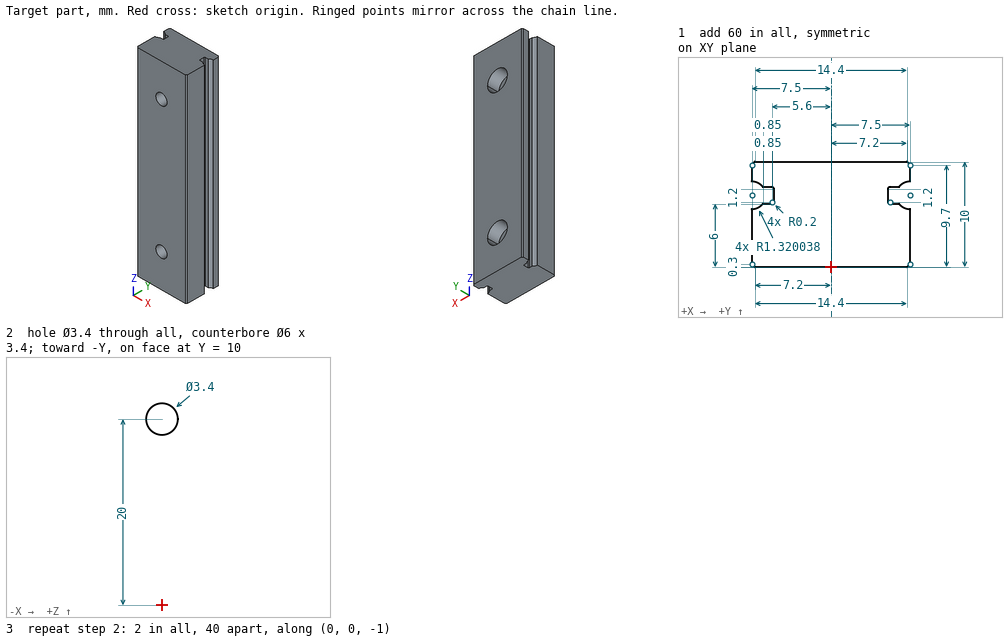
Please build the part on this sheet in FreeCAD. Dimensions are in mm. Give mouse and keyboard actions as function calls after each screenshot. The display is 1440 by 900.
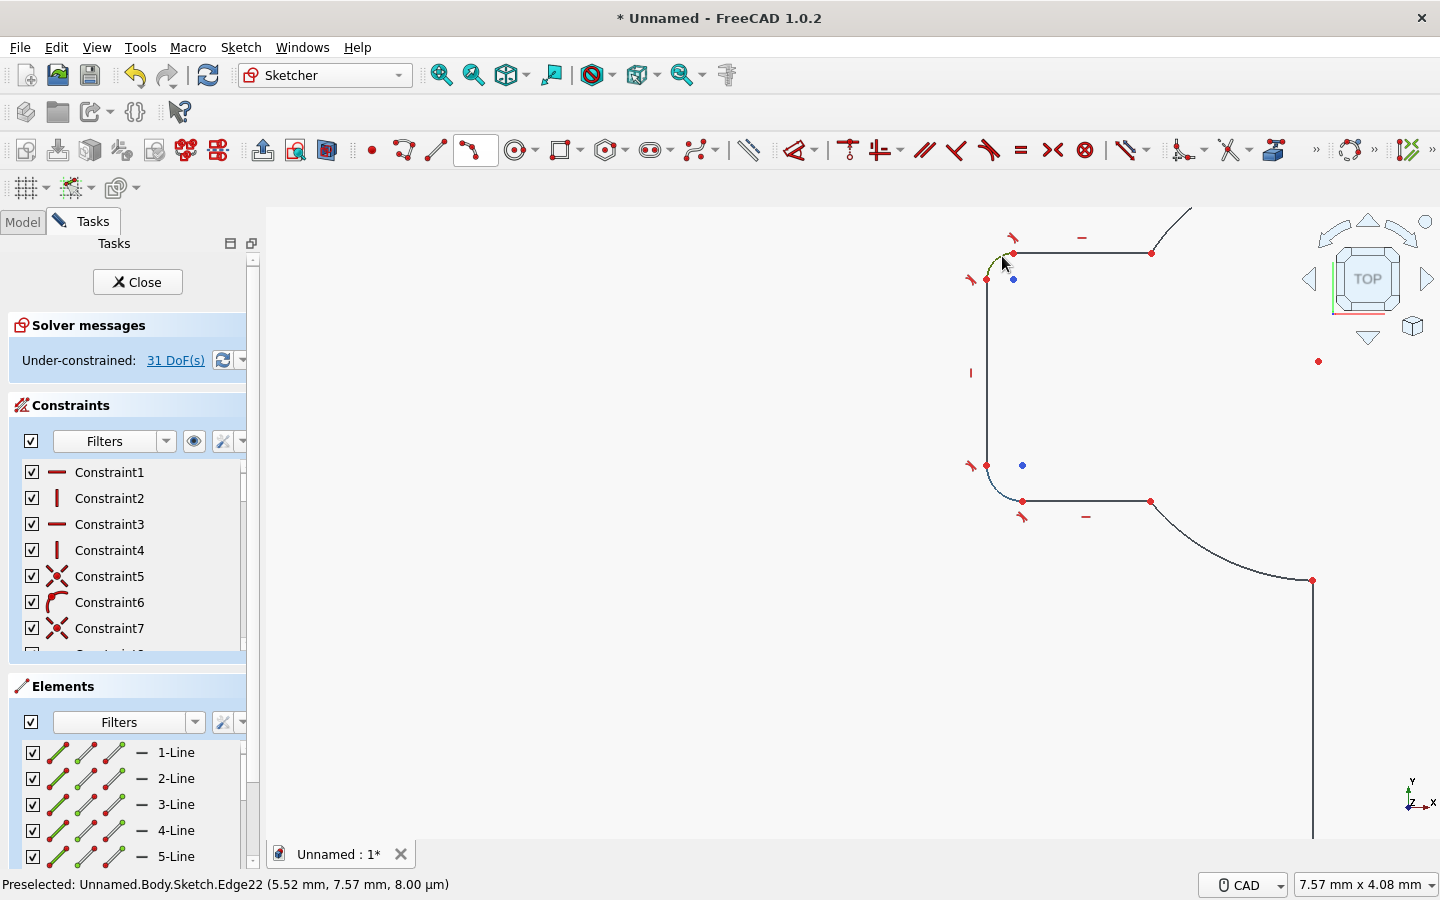
key(e)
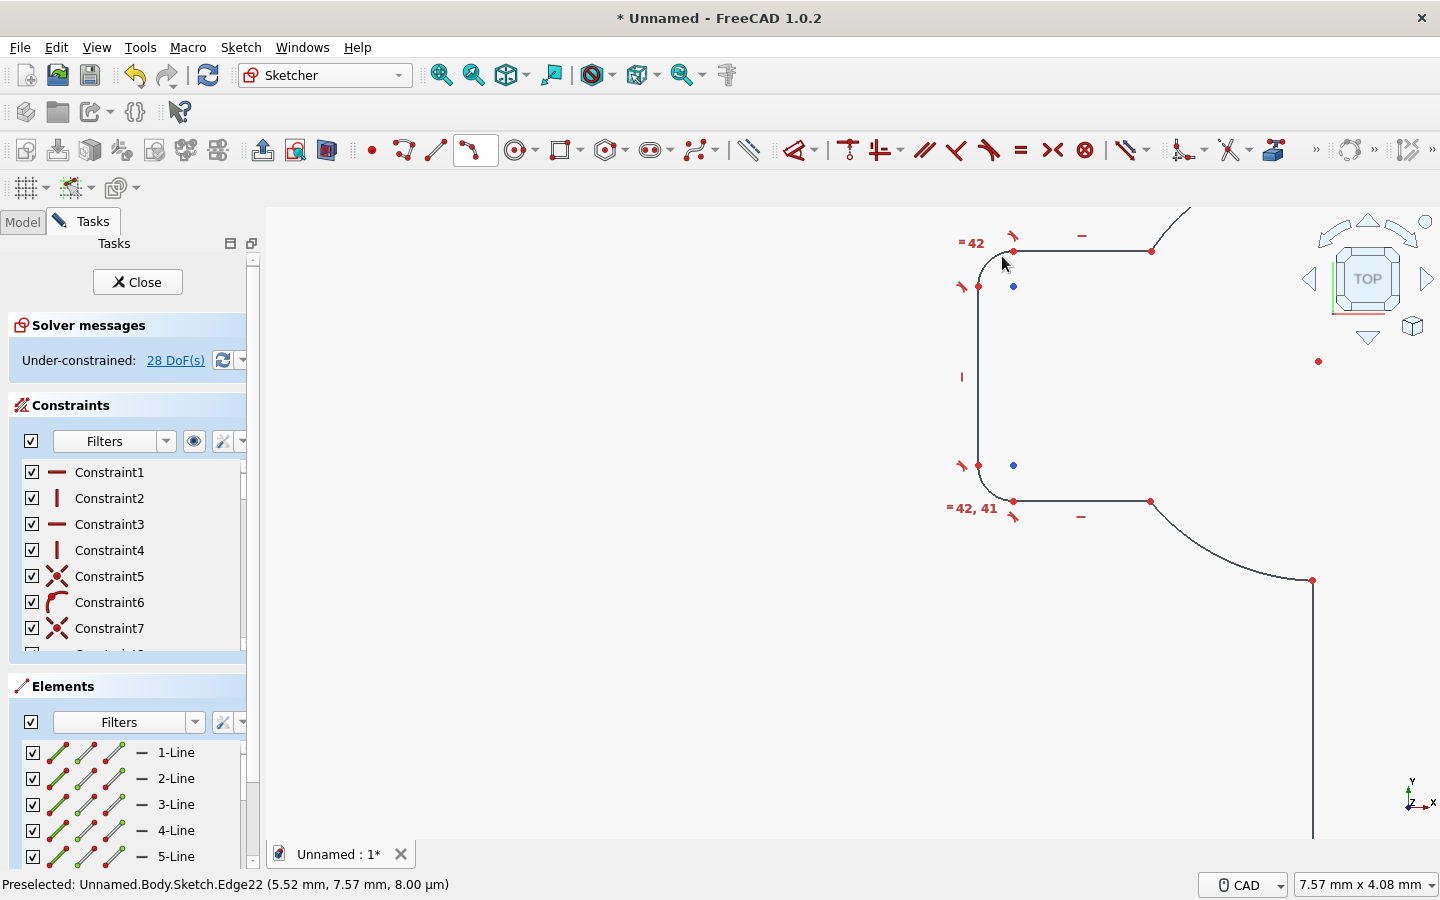
scroll(992, 481, down, 7)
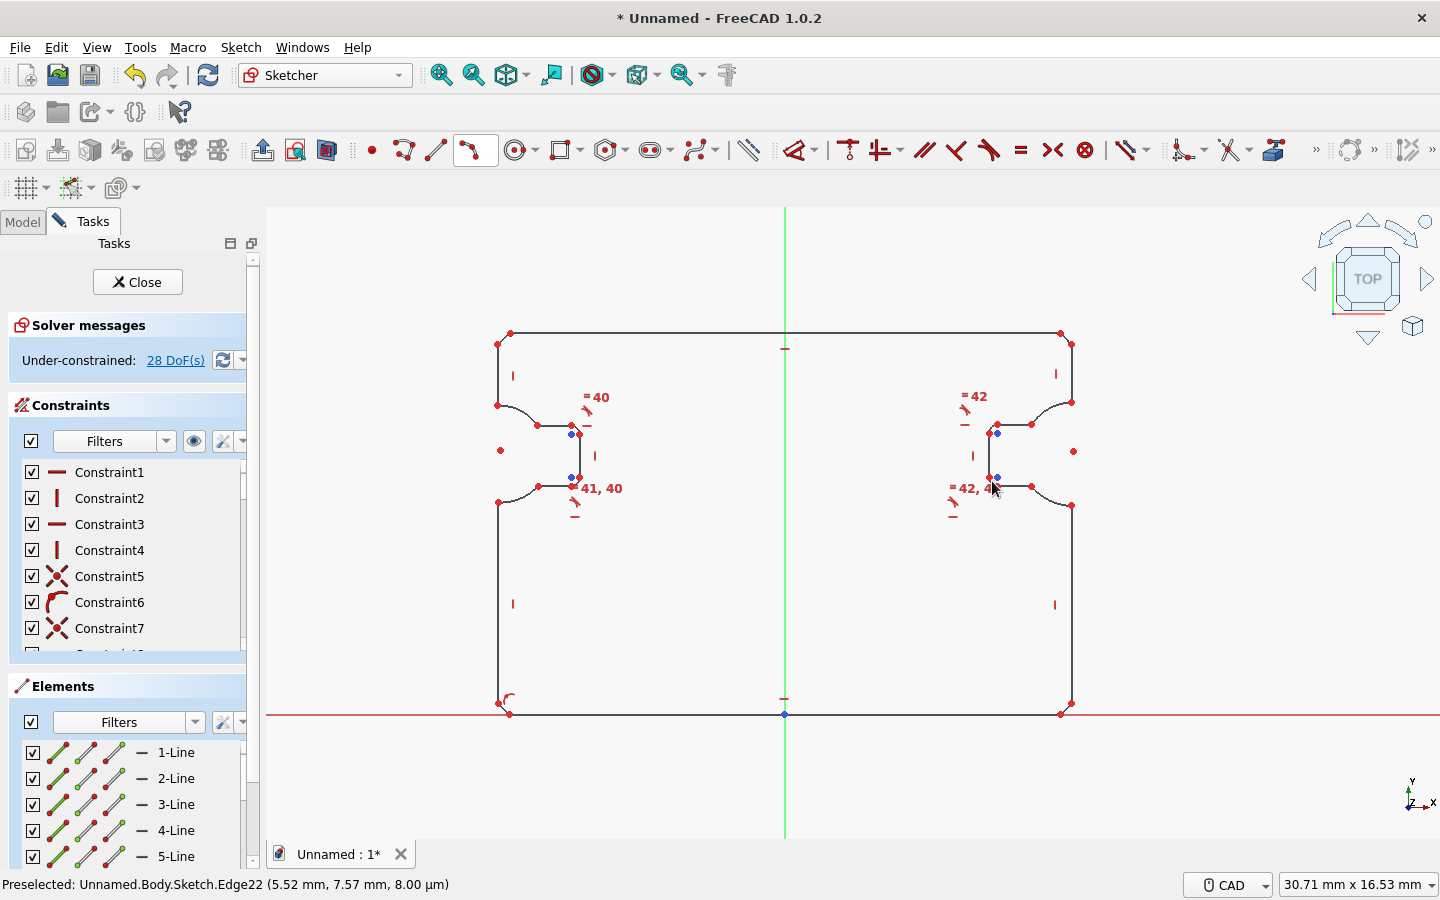
click(511, 501)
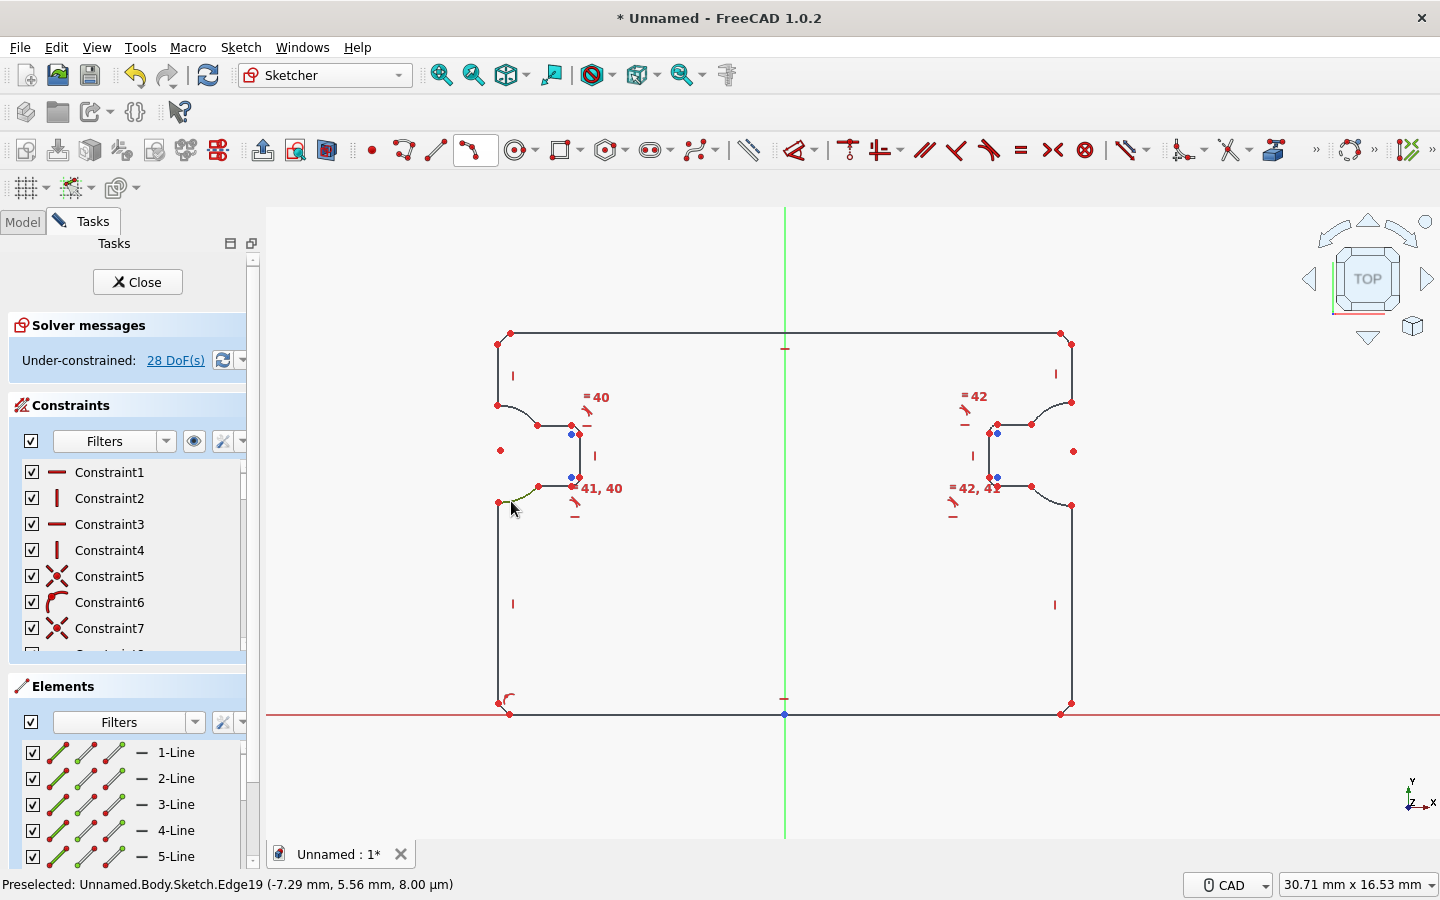
click(1041, 496)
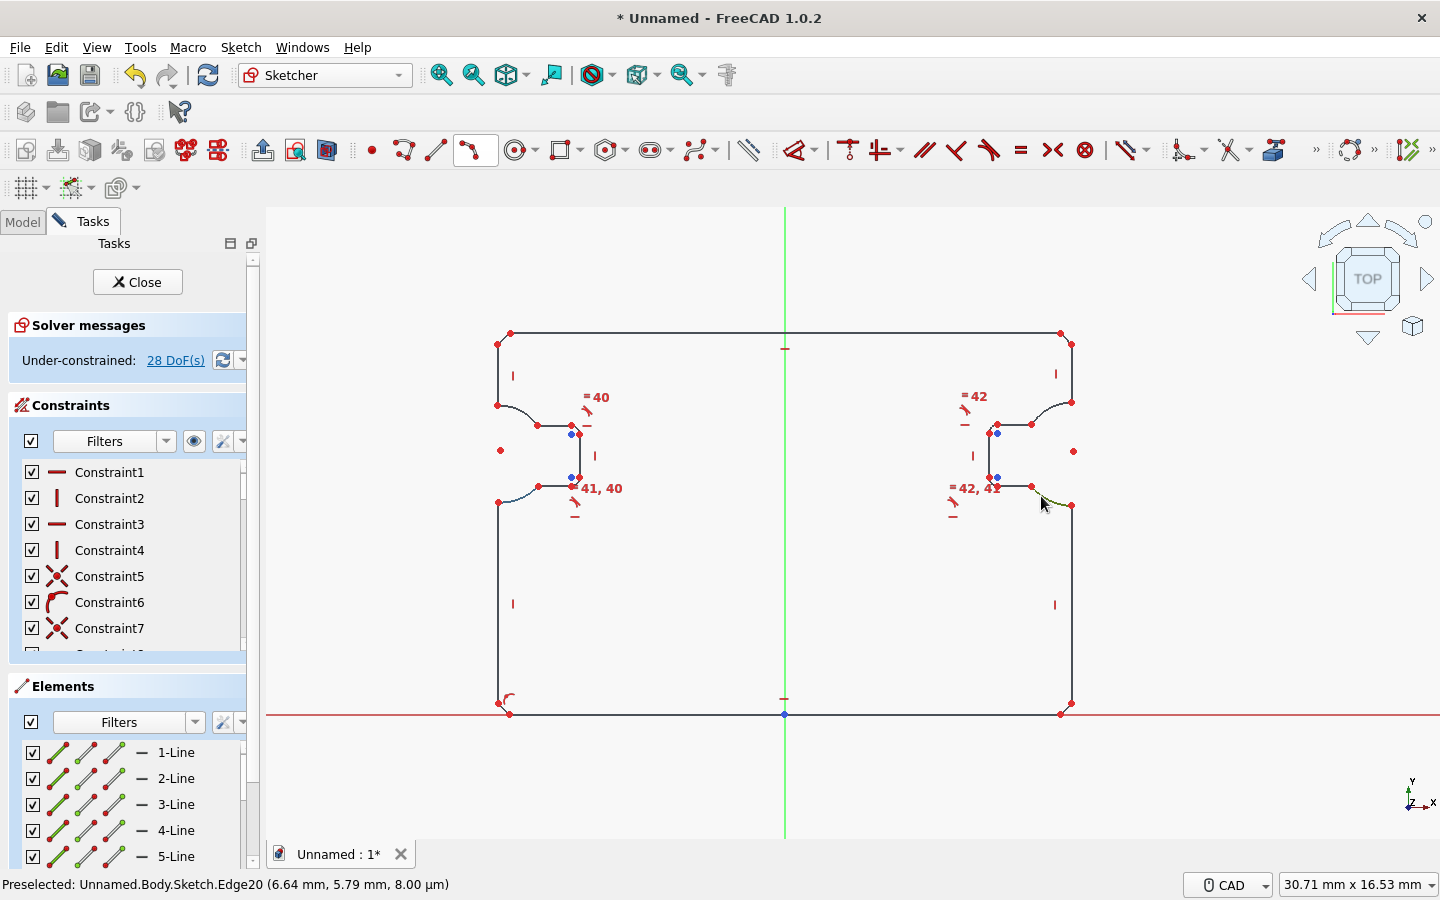
click(1058, 405)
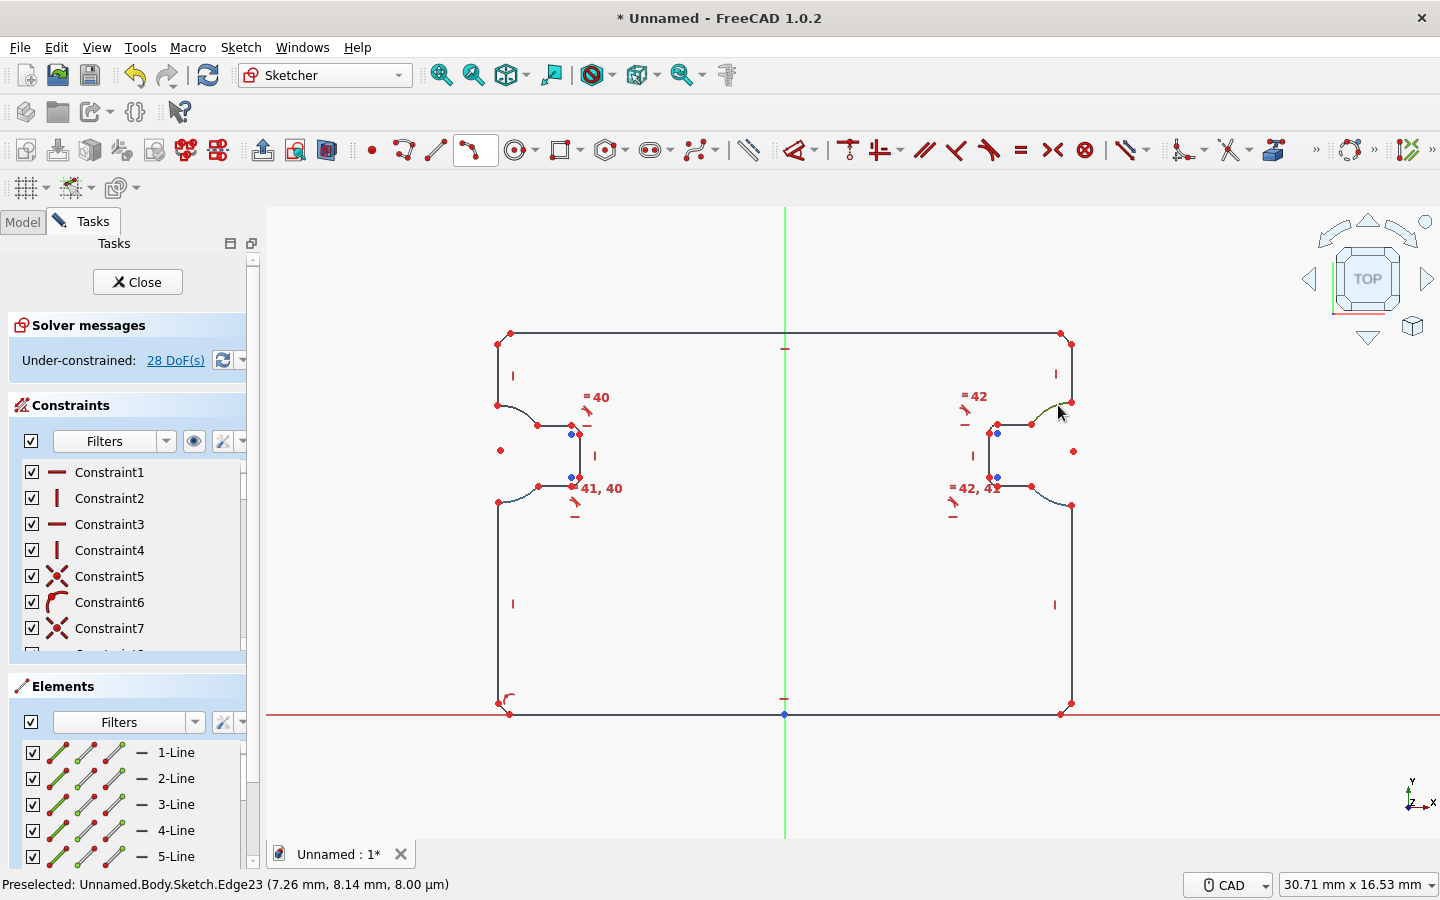
click(528, 415)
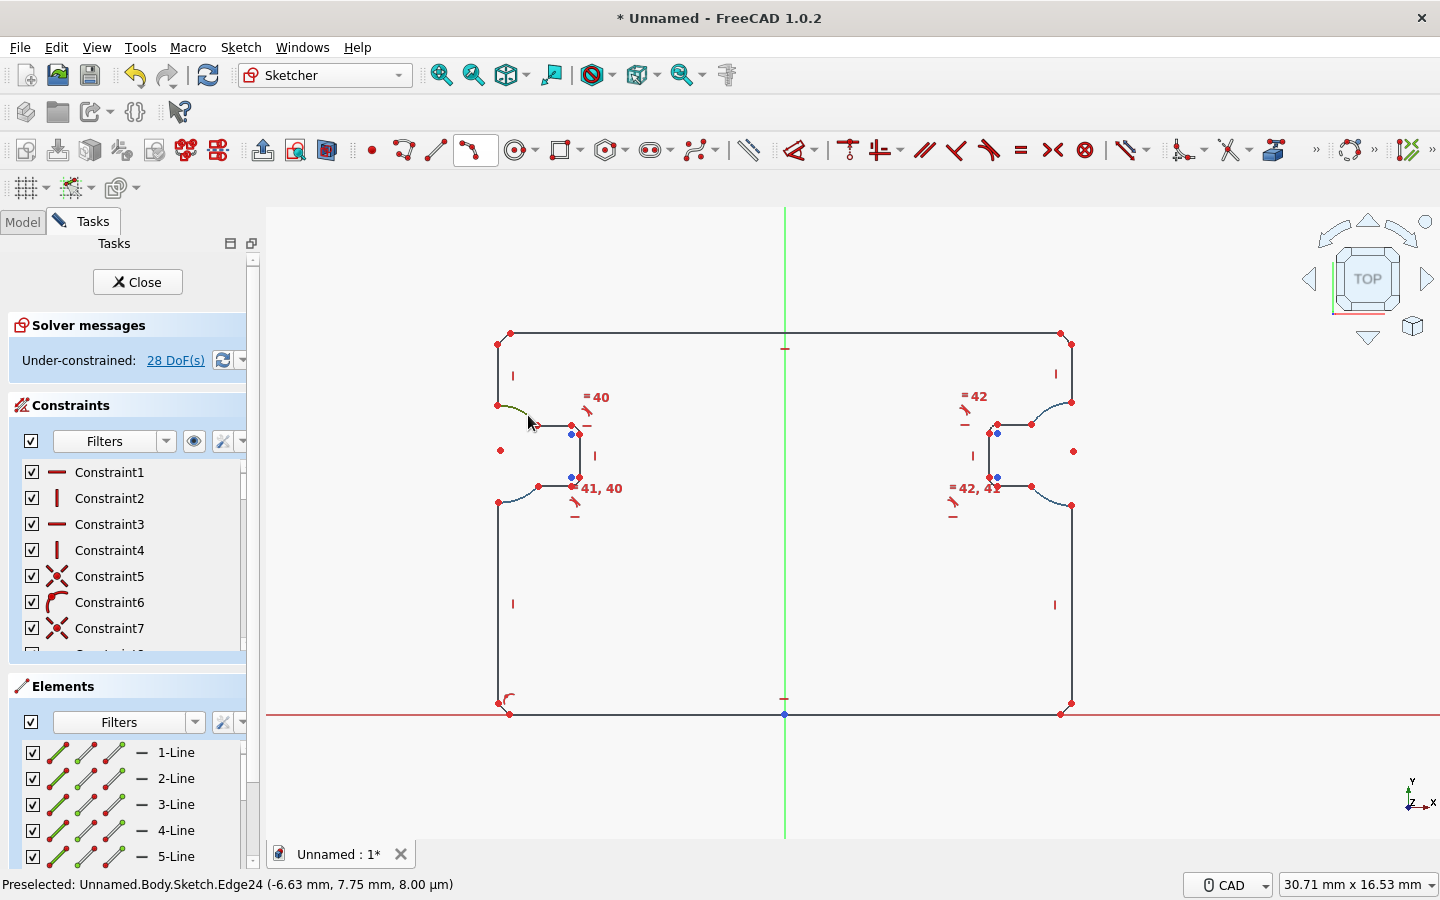
click(1022, 150)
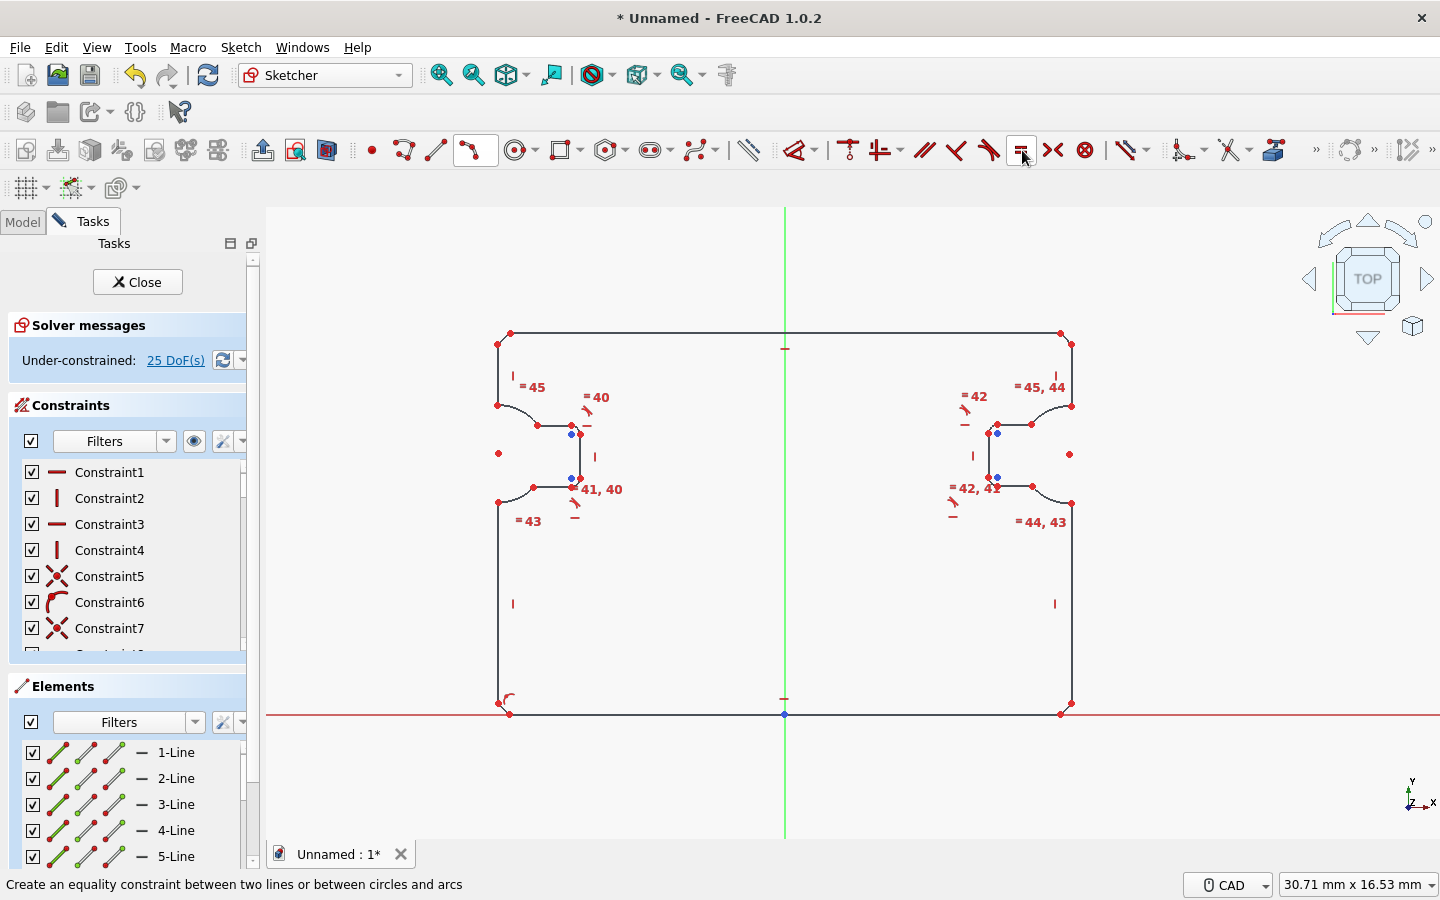
click(498, 454)